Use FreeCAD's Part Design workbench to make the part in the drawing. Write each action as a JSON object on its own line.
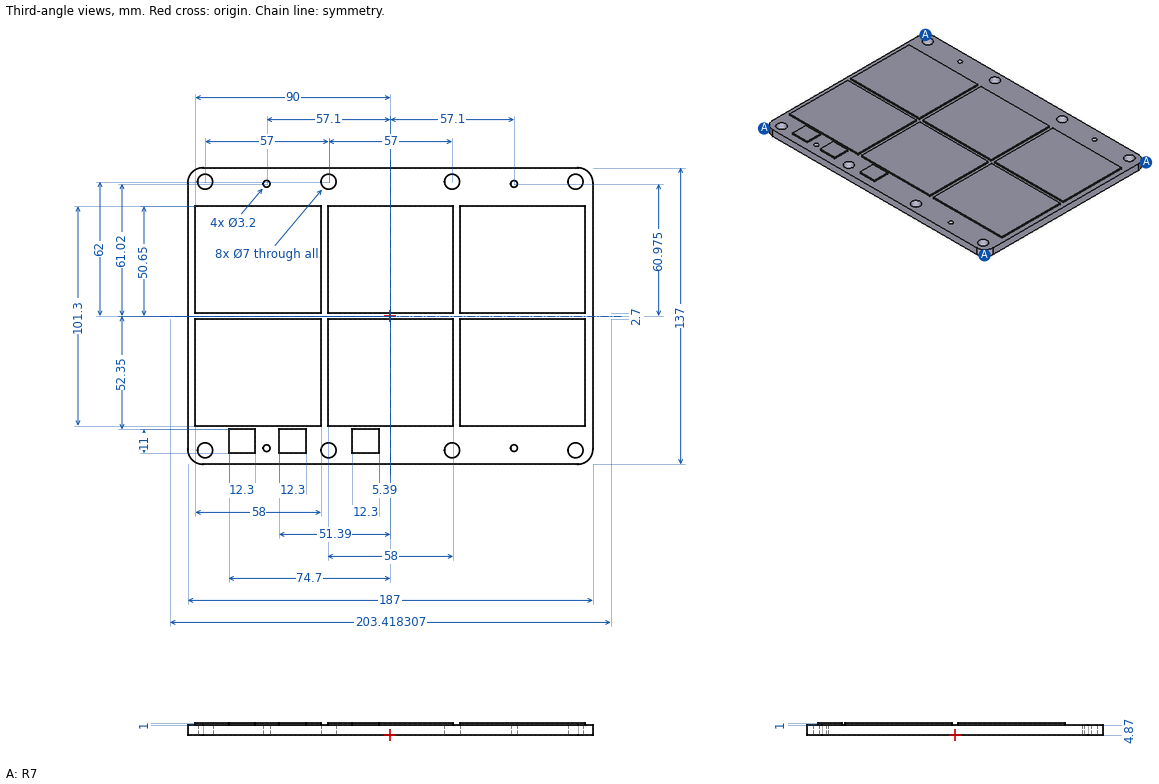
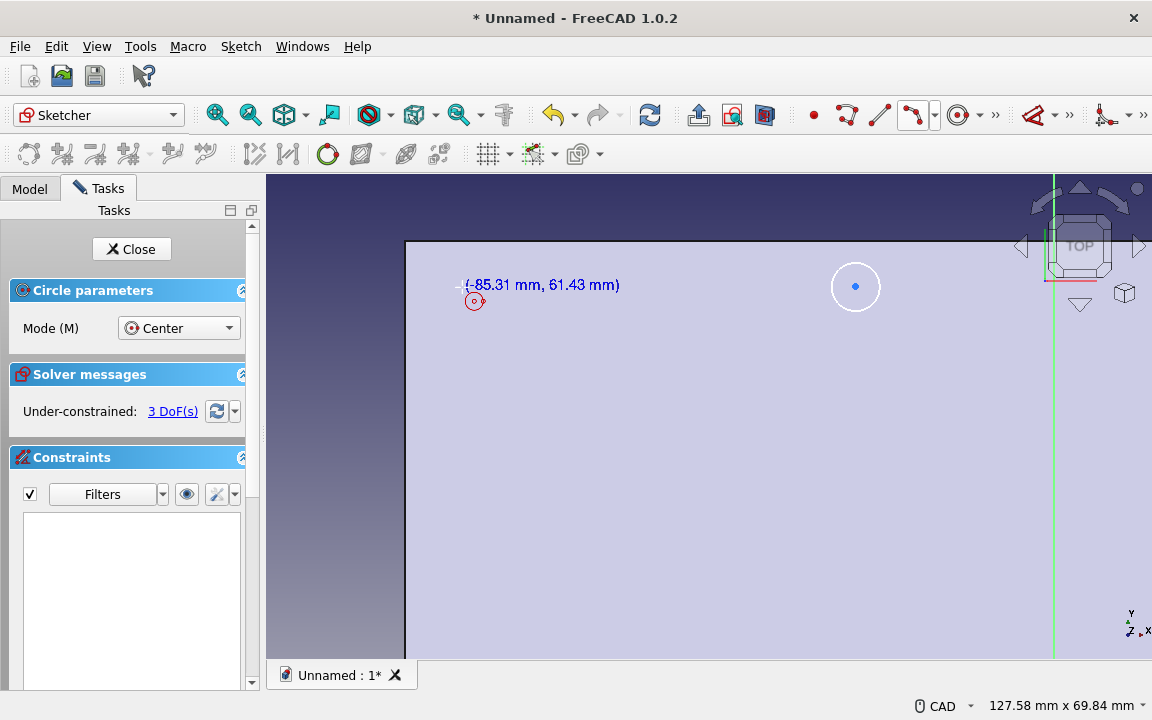
{"action": "left_click", "coordinate": [460, 286]}
{"action": "left_click", "coordinate": [477, 269]}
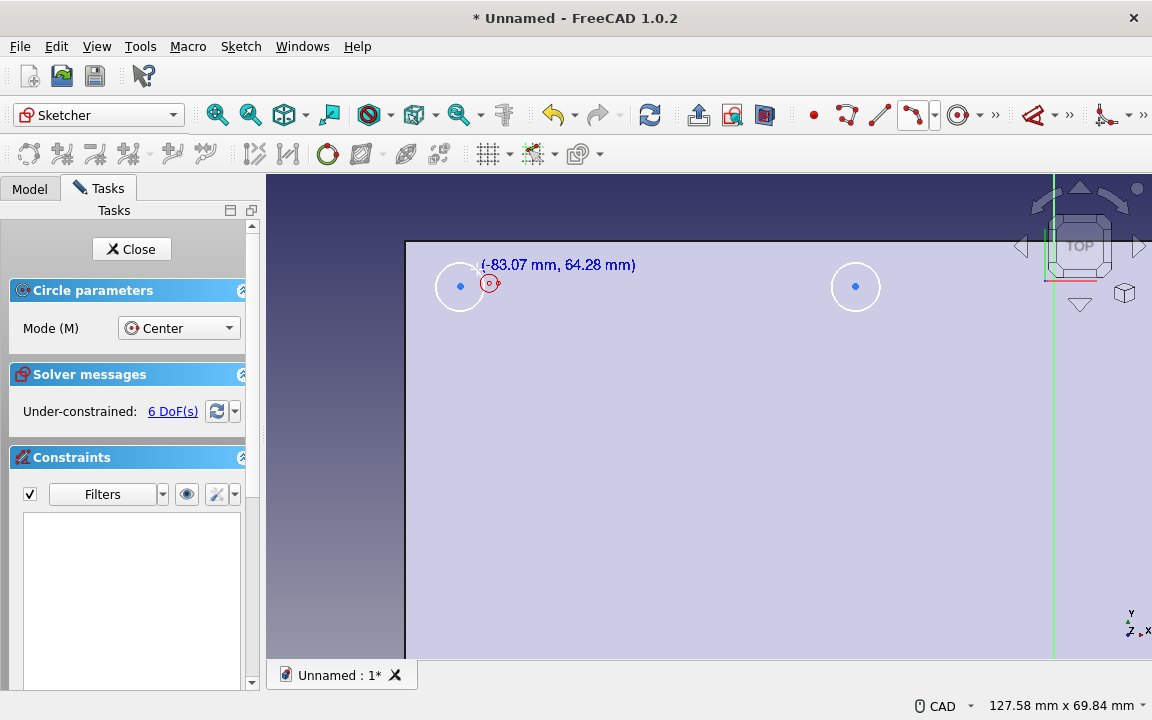
{"action": "scroll", "coordinate": [462, 287], "scroll_direction": "down", "scroll_amount": 6}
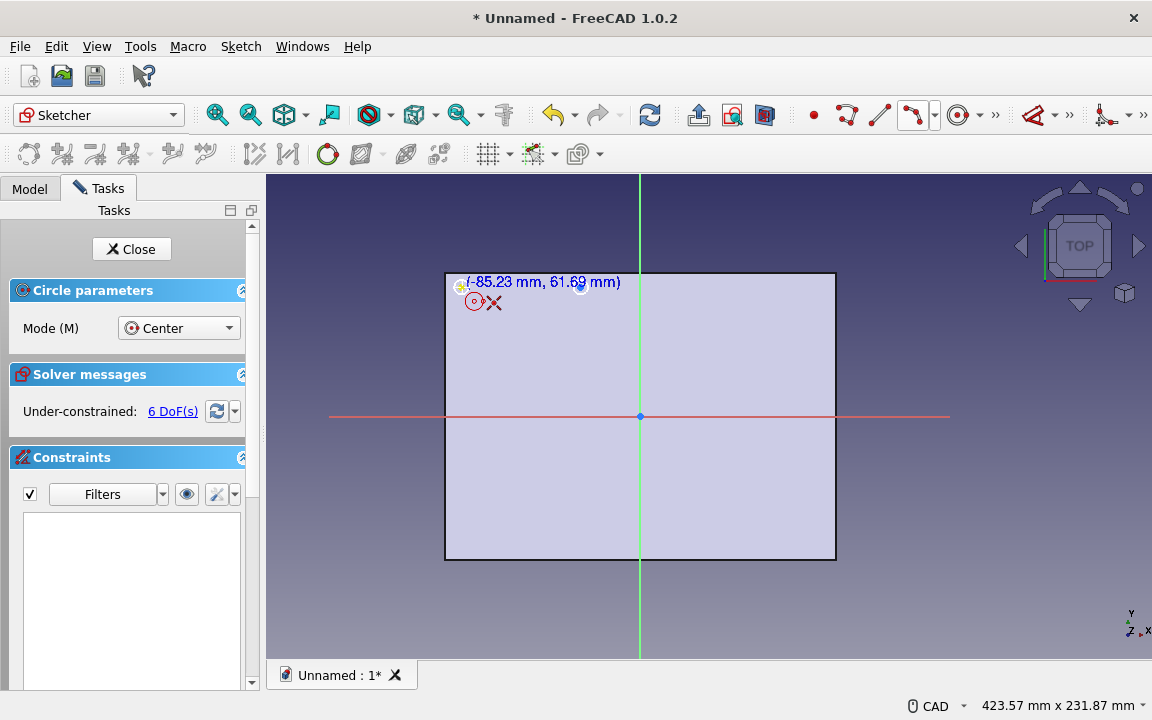
{"action": "scroll", "coordinate": [700, 287], "scroll_direction": "up", "scroll_amount": 6}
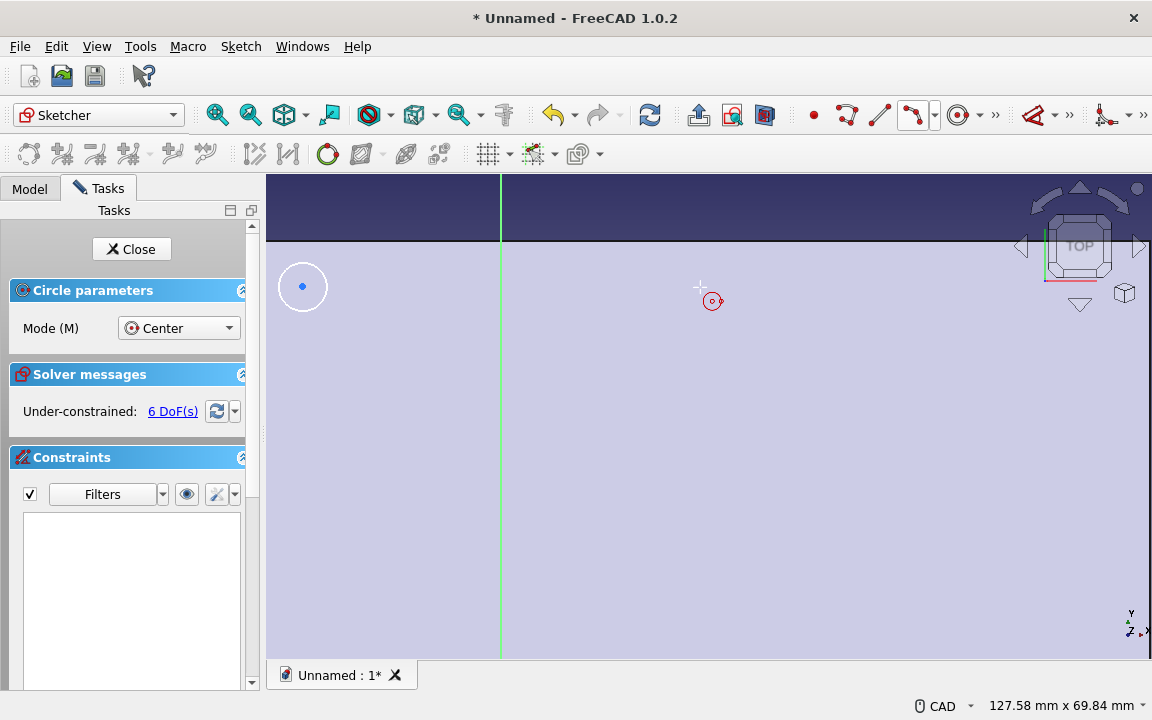
{"action": "left_click", "coordinate": [699, 286]}
{"action": "left_click", "coordinate": [716, 269]}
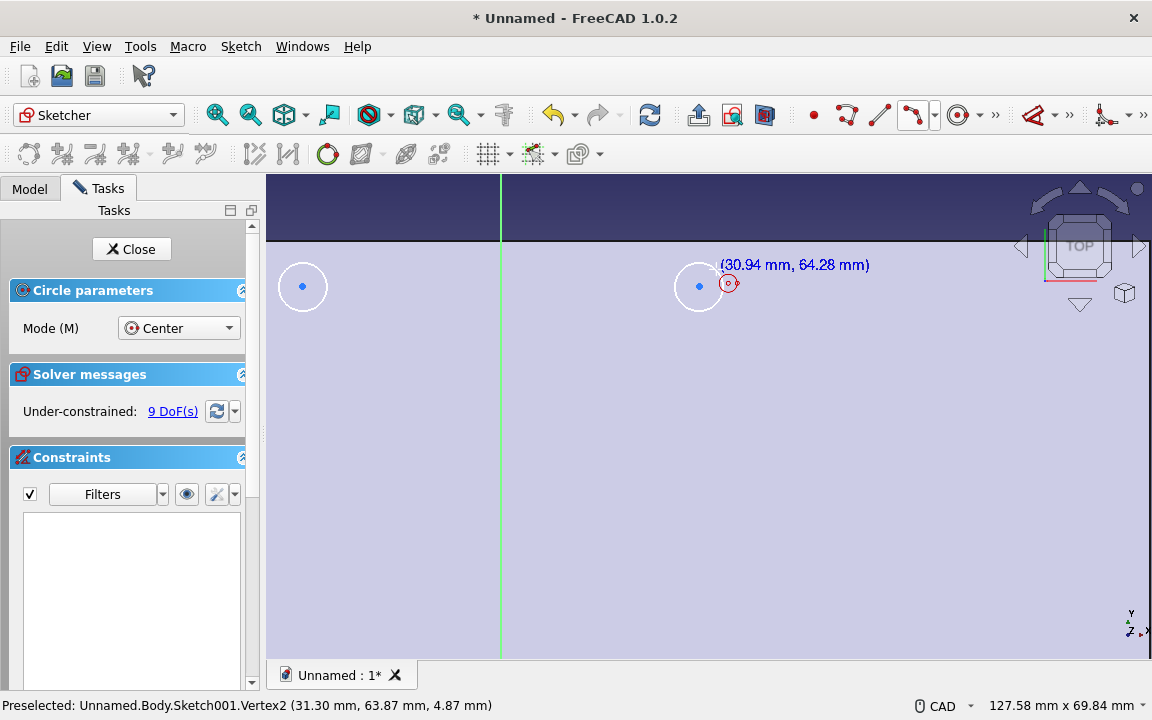
{"action": "scroll", "coordinate": [701, 287], "scroll_direction": "down", "scroll_amount": 6}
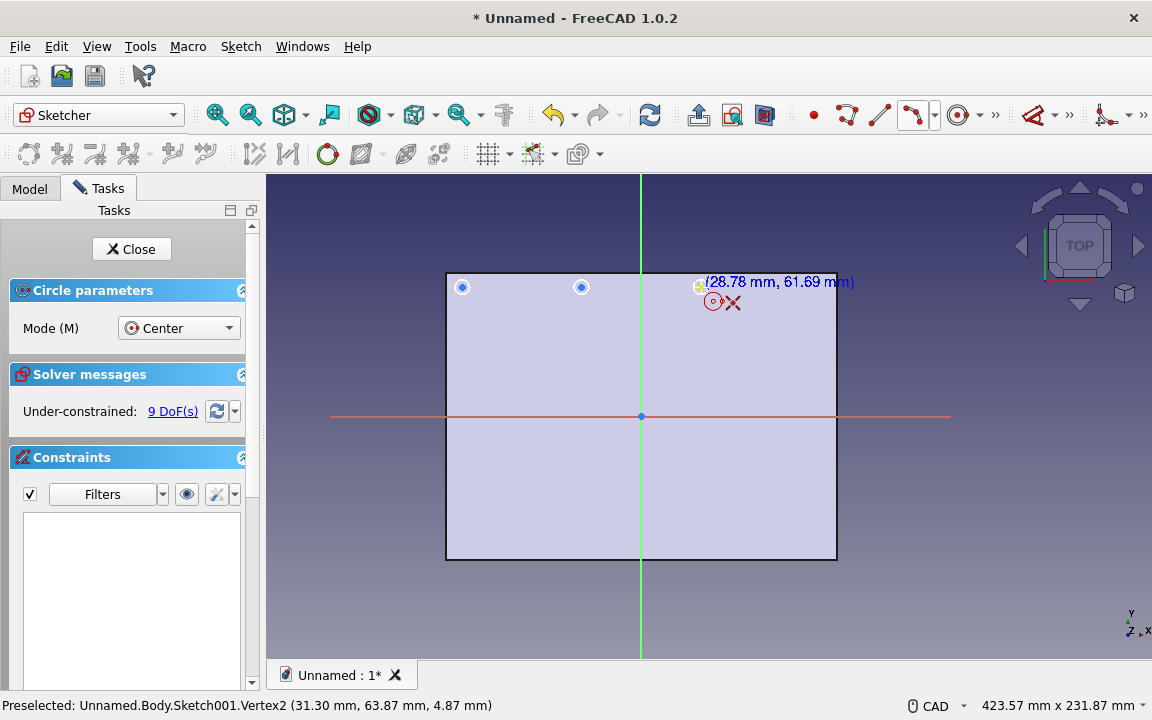
{"action": "scroll", "coordinate": [820, 287], "scroll_direction": "up", "scroll_amount": 6}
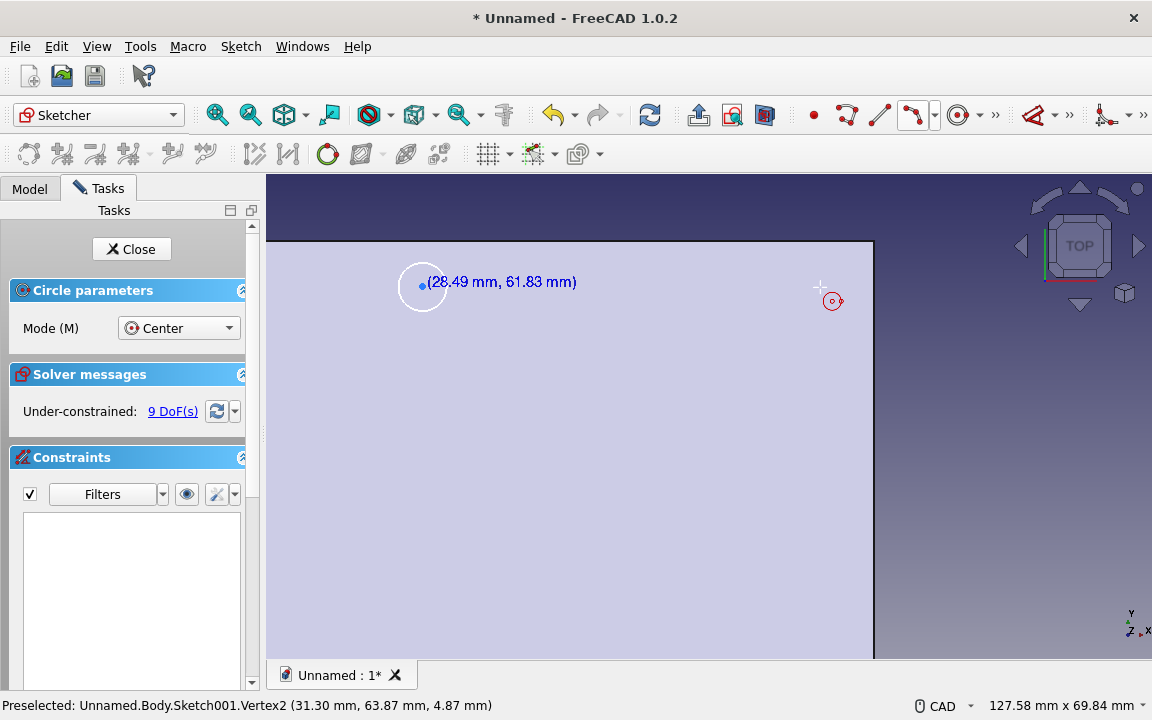
{"action": "left_click", "coordinate": [818, 286]}
{"action": "left_click", "coordinate": [836, 269]}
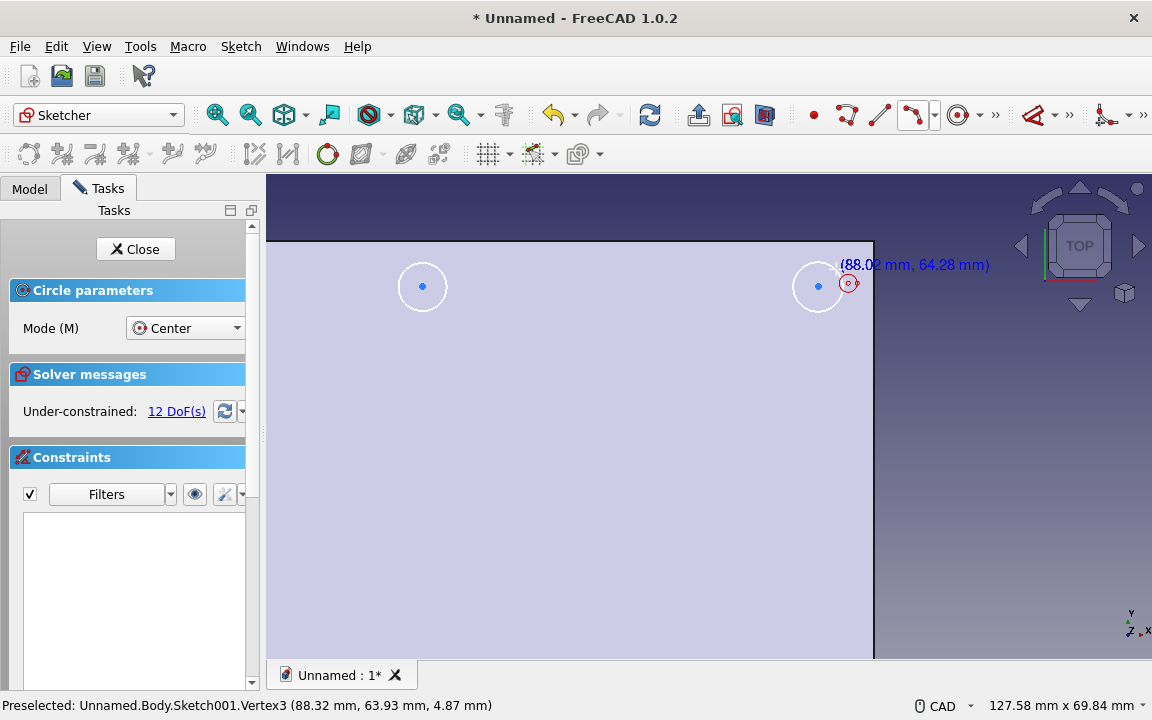
{"action": "scroll", "coordinate": [820, 287], "scroll_direction": "down", "scroll_amount": 6}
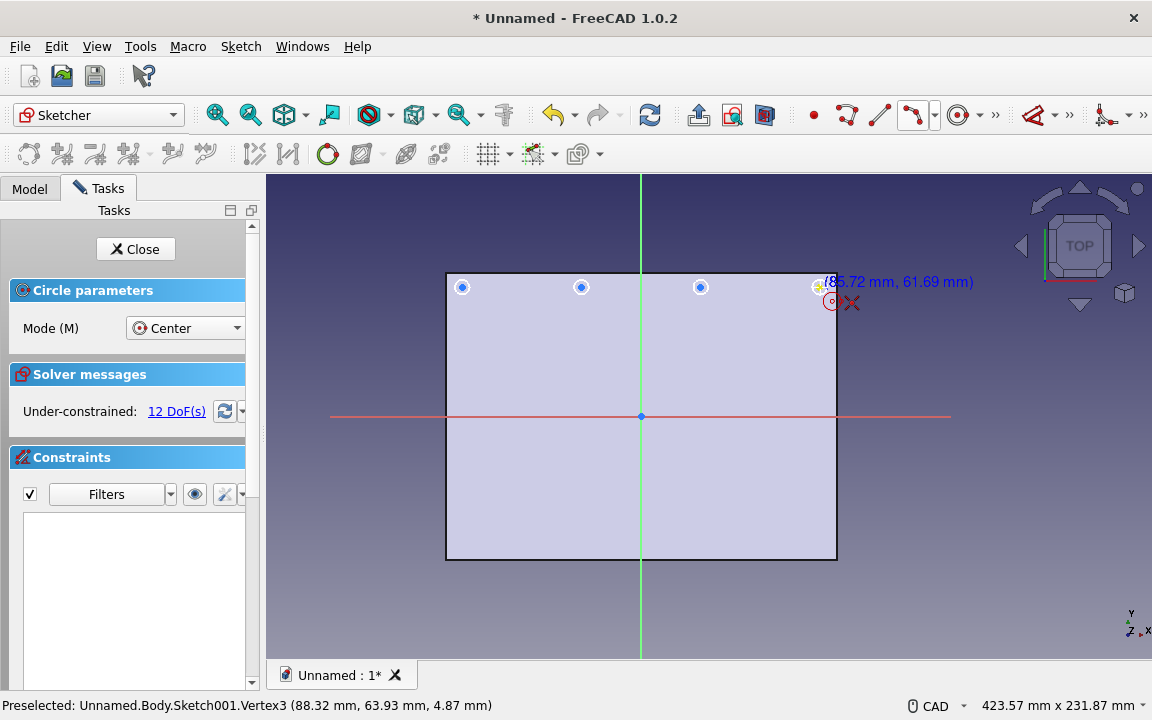
{"action": "scroll", "coordinate": [820, 546], "scroll_direction": "up", "scroll_amount": 6}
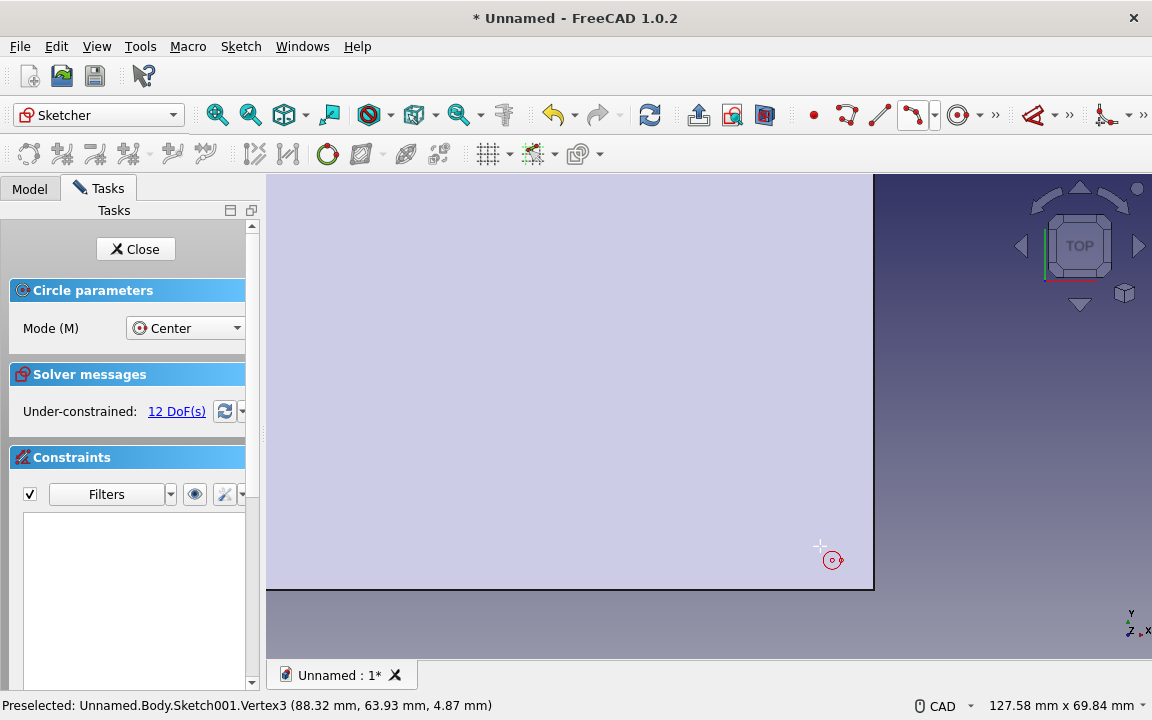
{"action": "left_click", "coordinate": [818, 545]}
{"action": "left_click", "coordinate": [836, 528]}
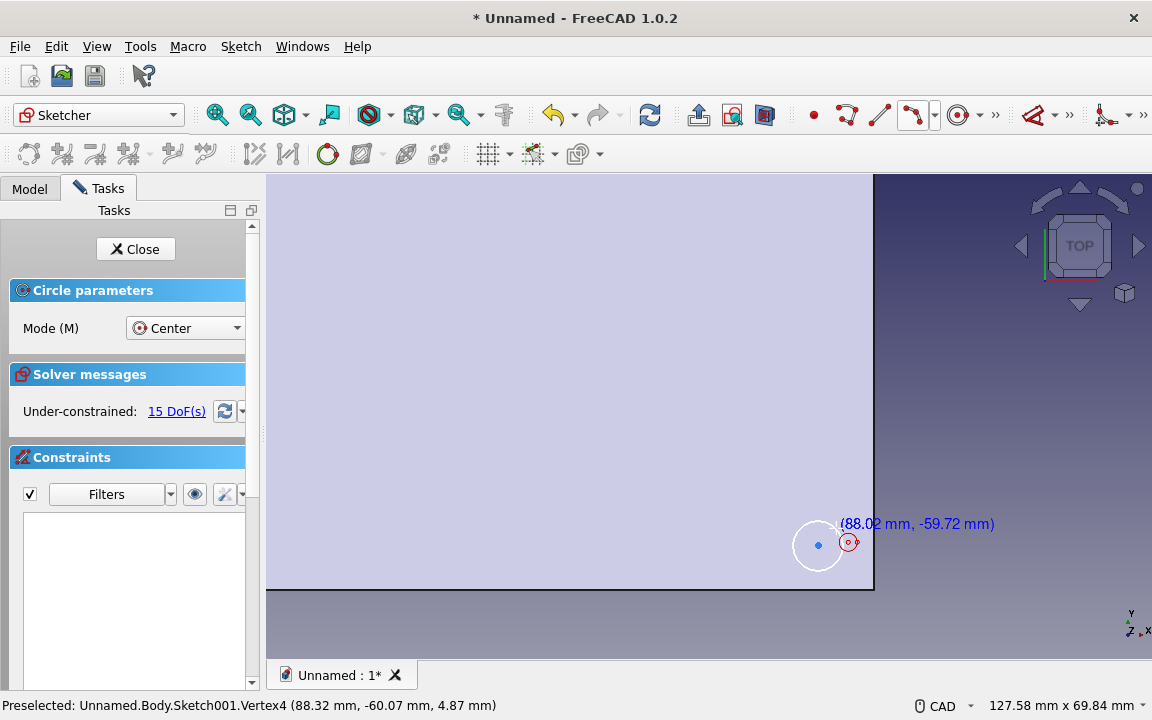
{"action": "left_click", "coordinate": [423, 545]}
{"action": "left_click", "coordinate": [440, 528]}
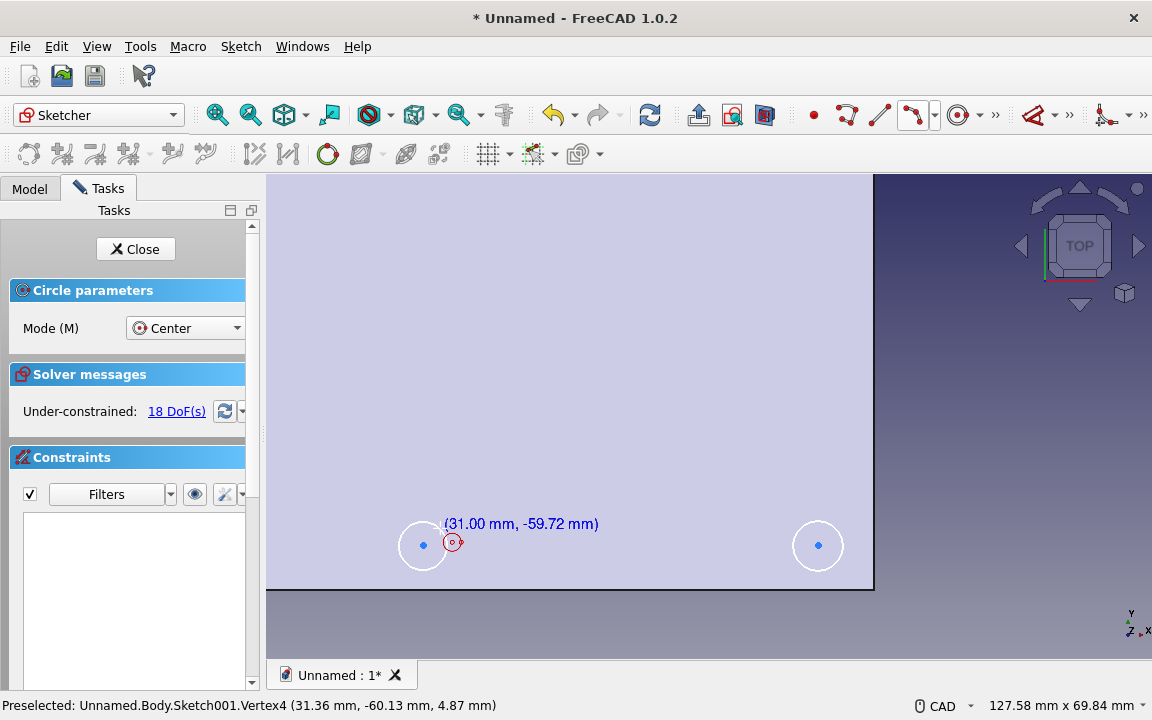
{"action": "scroll", "coordinate": [820, 547], "scroll_direction": "down", "scroll_amount": 6}